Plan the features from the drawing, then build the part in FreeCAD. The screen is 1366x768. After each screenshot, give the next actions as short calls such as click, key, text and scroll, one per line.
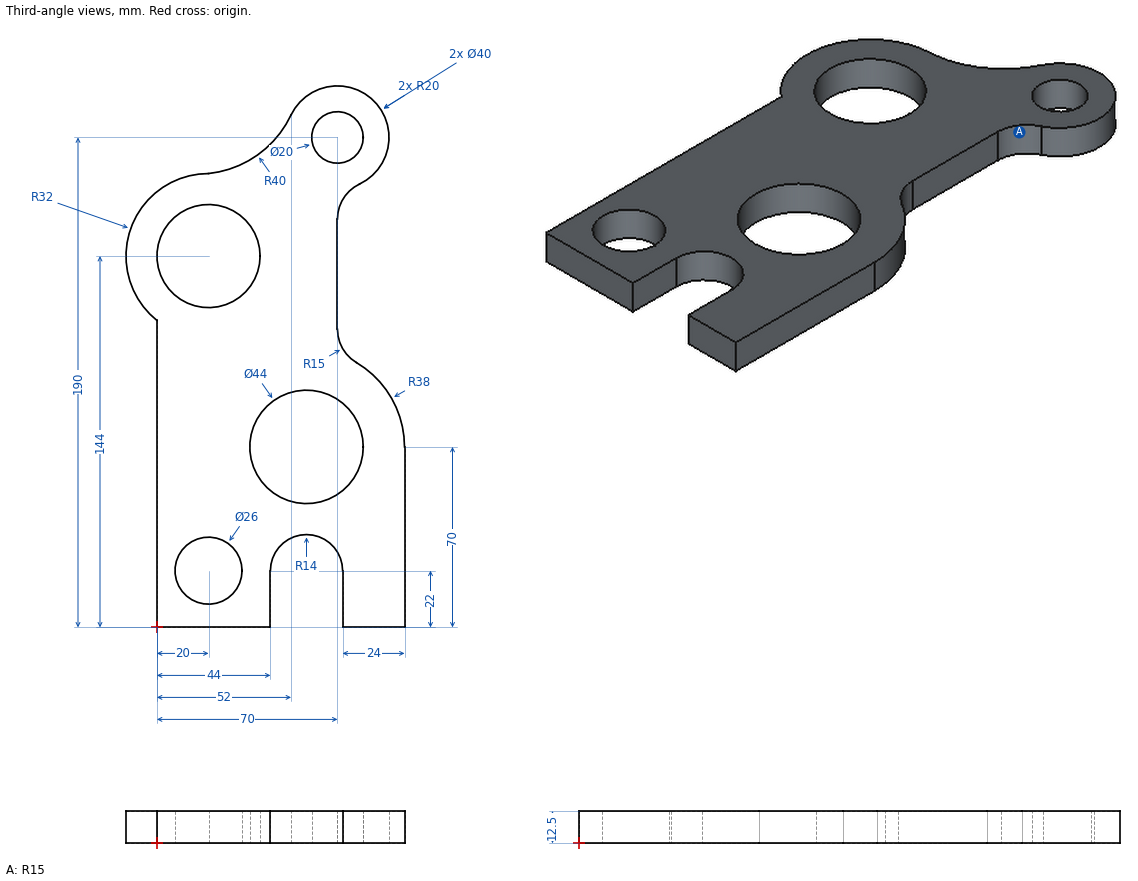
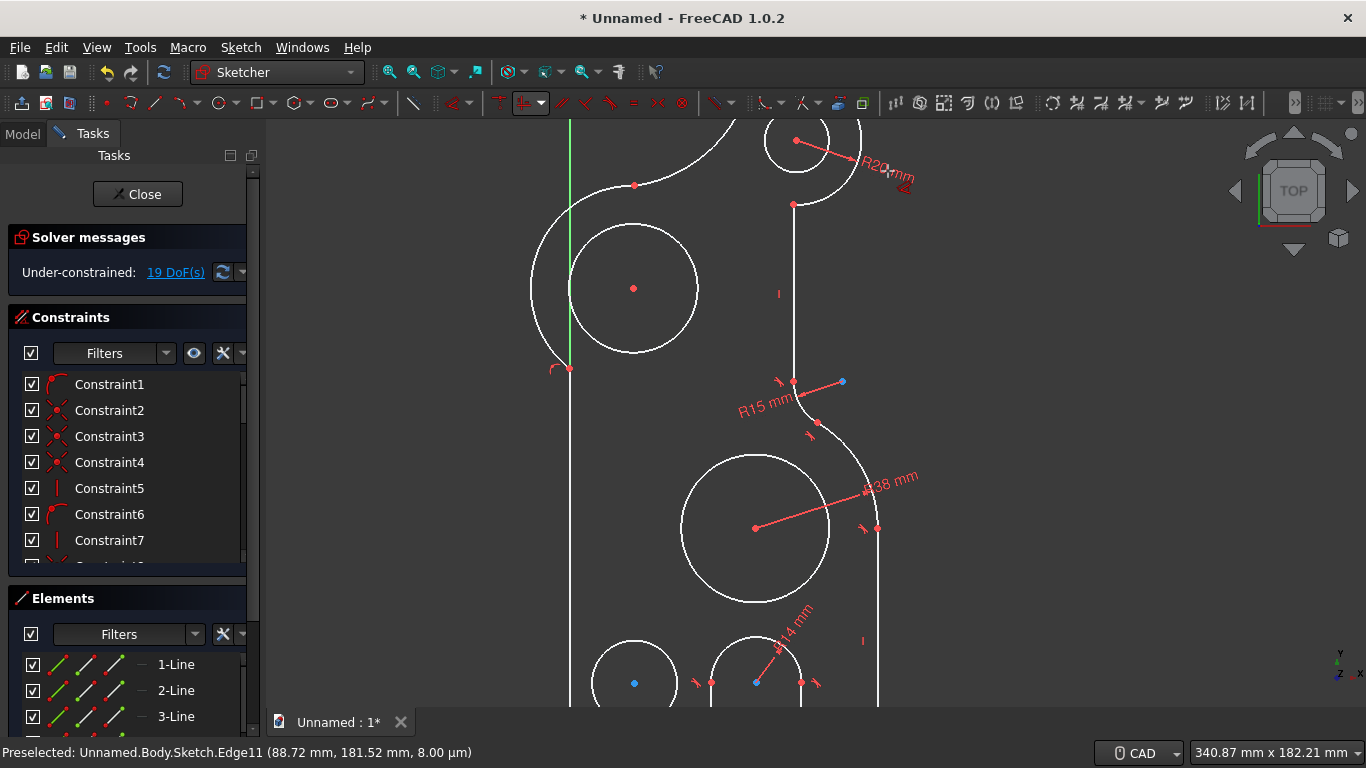
click(672, 175)
click(685, 204)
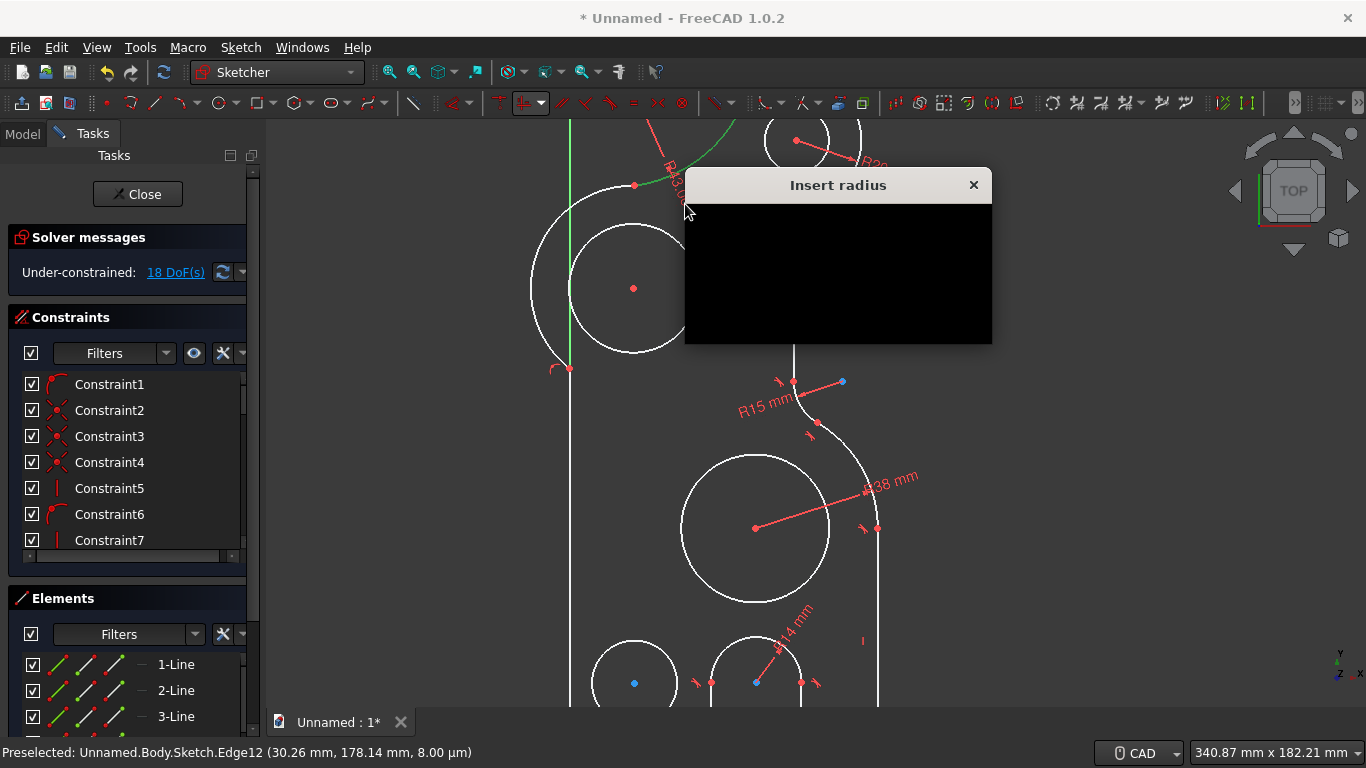
text(40)
key(Return)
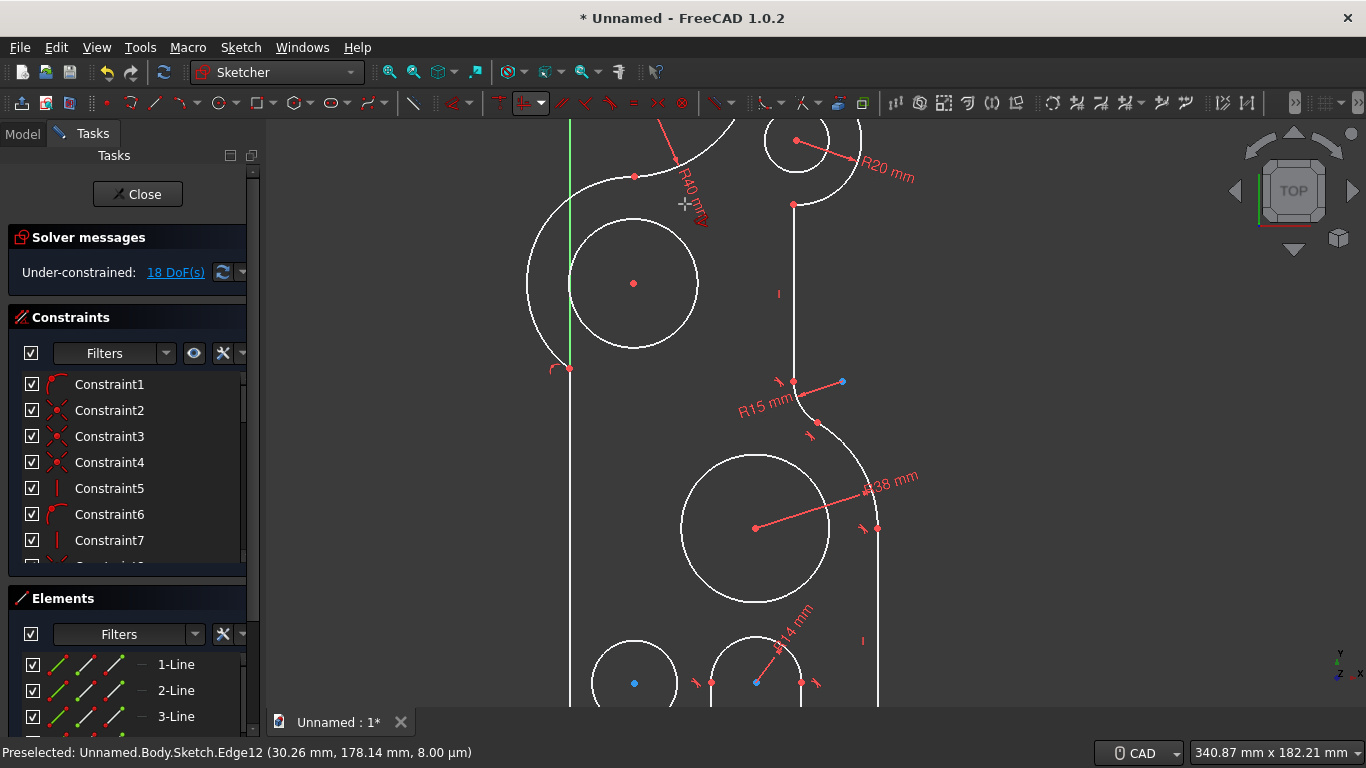
click(529, 302)
click(497, 308)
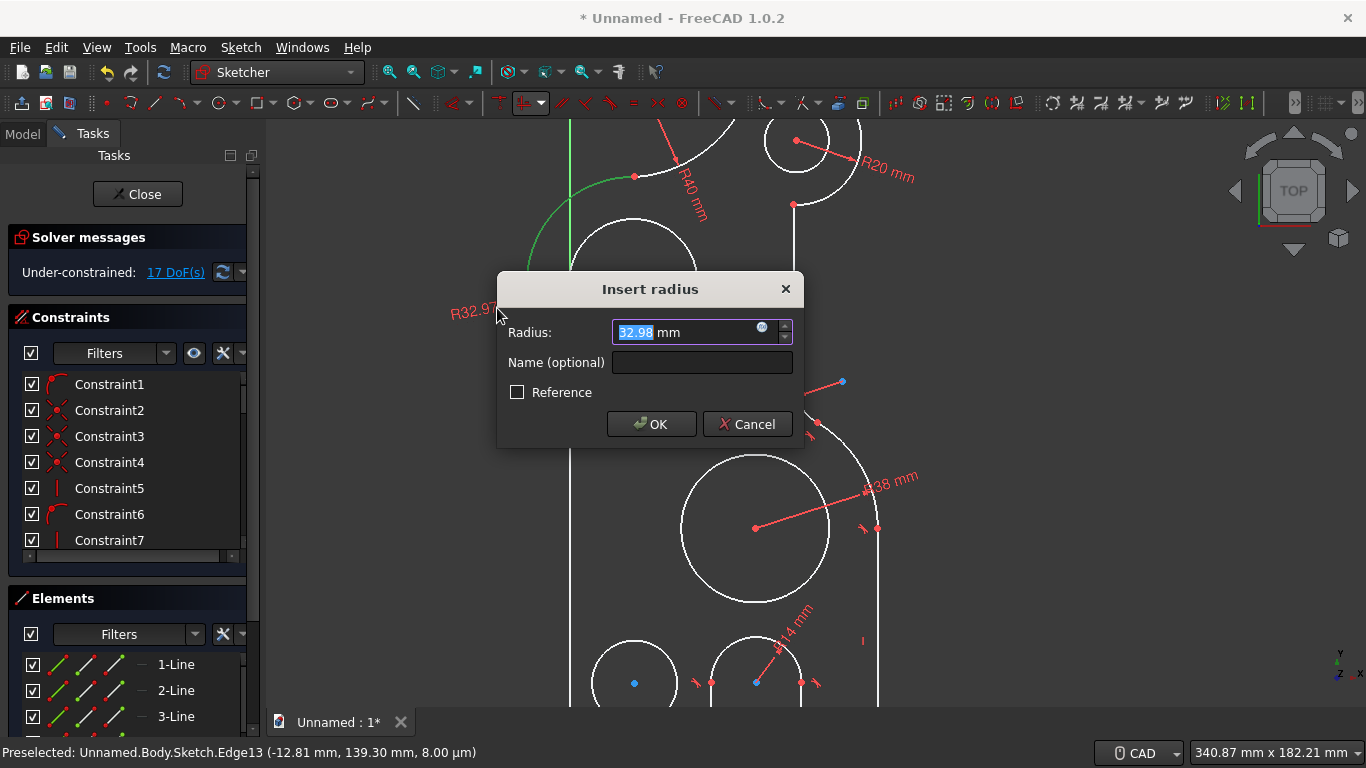
text(32)
key(Return)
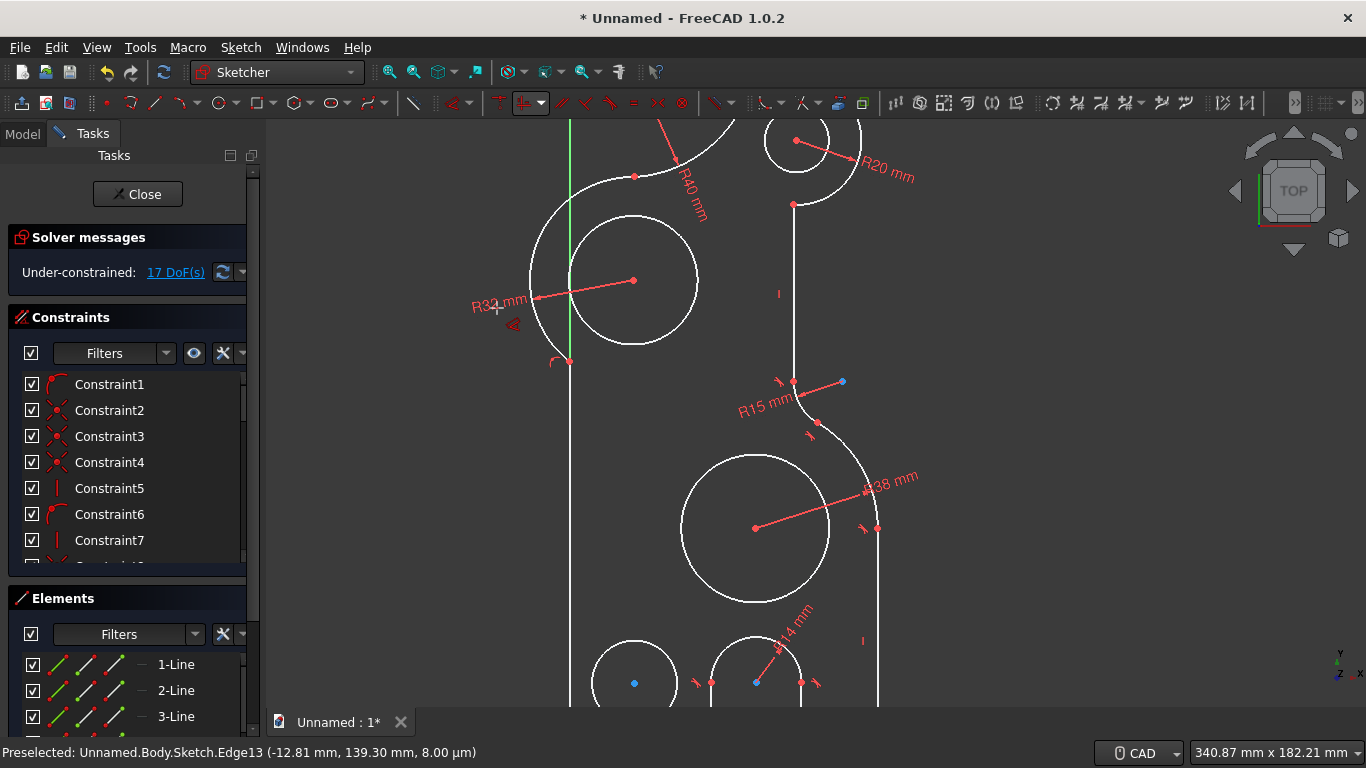
click(665, 653)
click(688, 630)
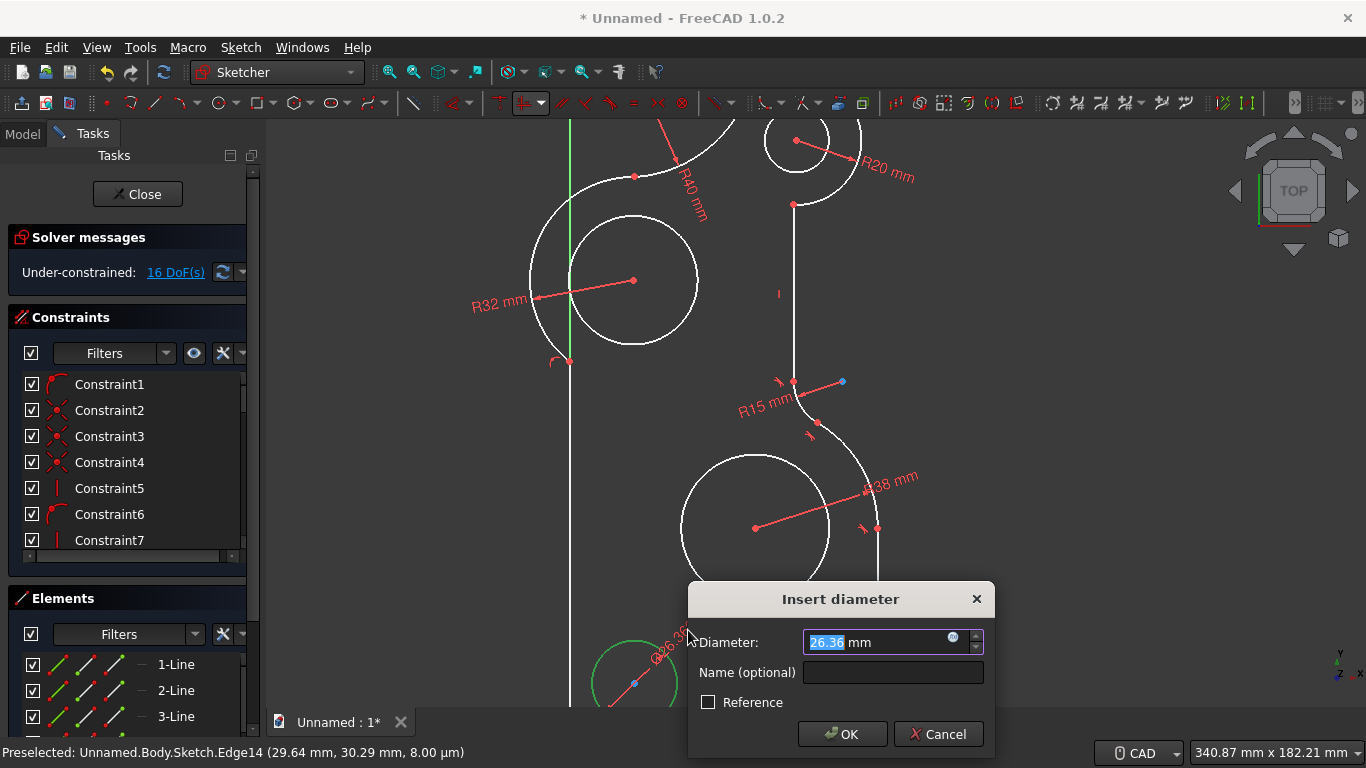
text(26)
key(Return)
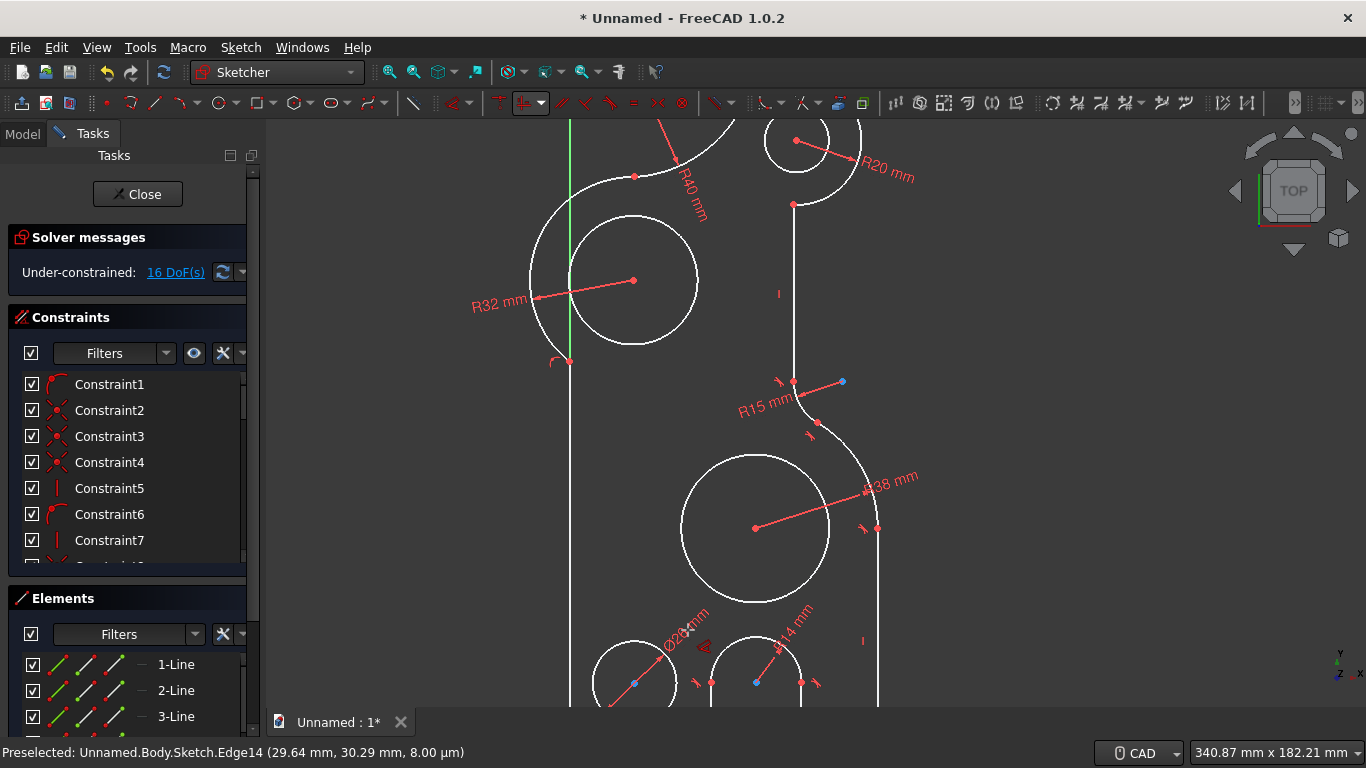
click(807, 476)
click(829, 453)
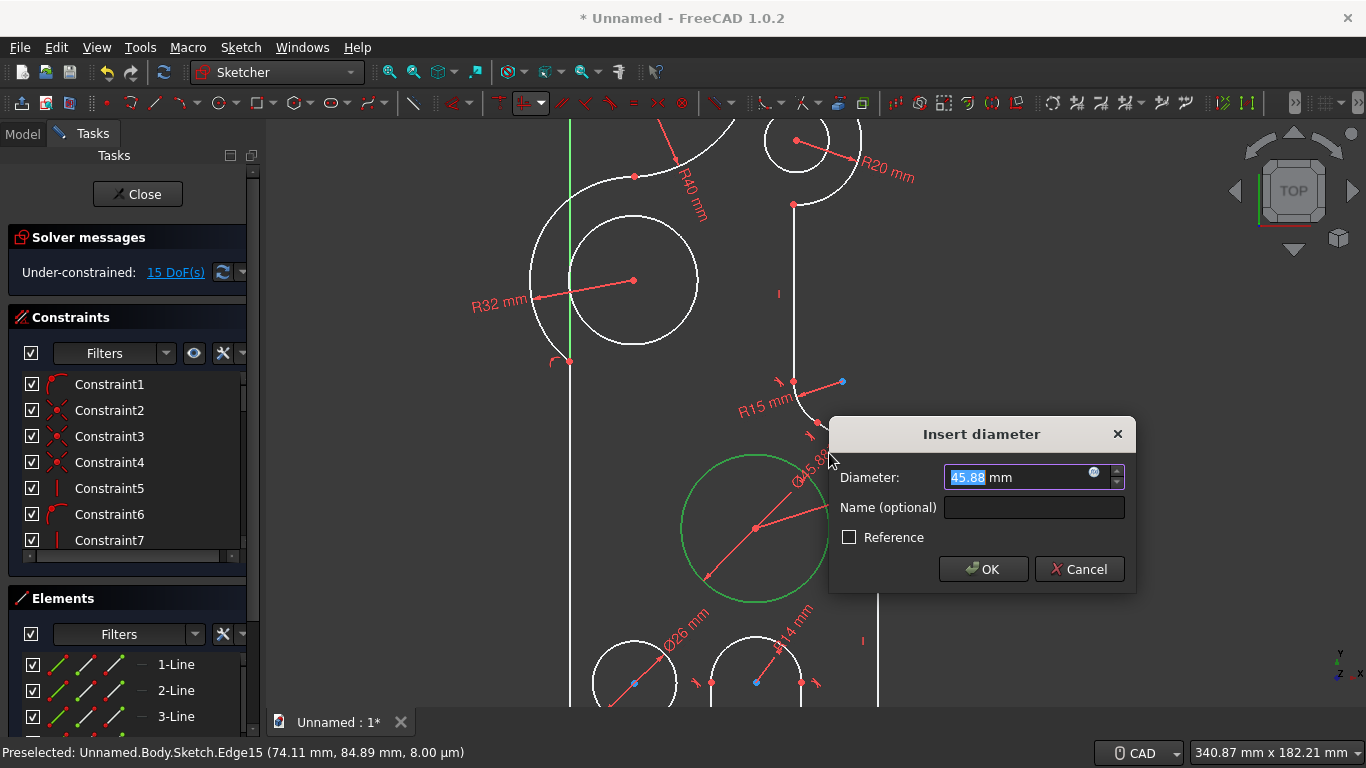
text(44)
key(Return)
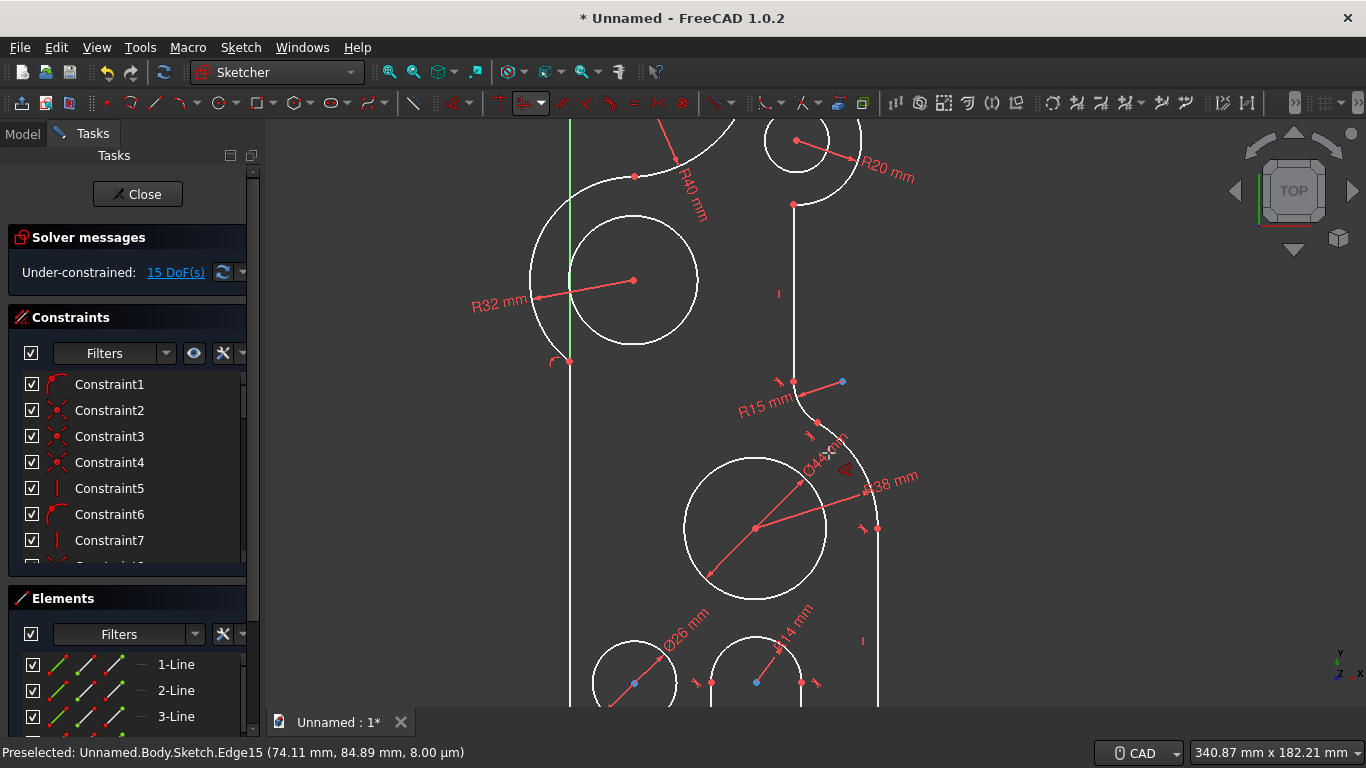
click(679, 235)
click(726, 254)